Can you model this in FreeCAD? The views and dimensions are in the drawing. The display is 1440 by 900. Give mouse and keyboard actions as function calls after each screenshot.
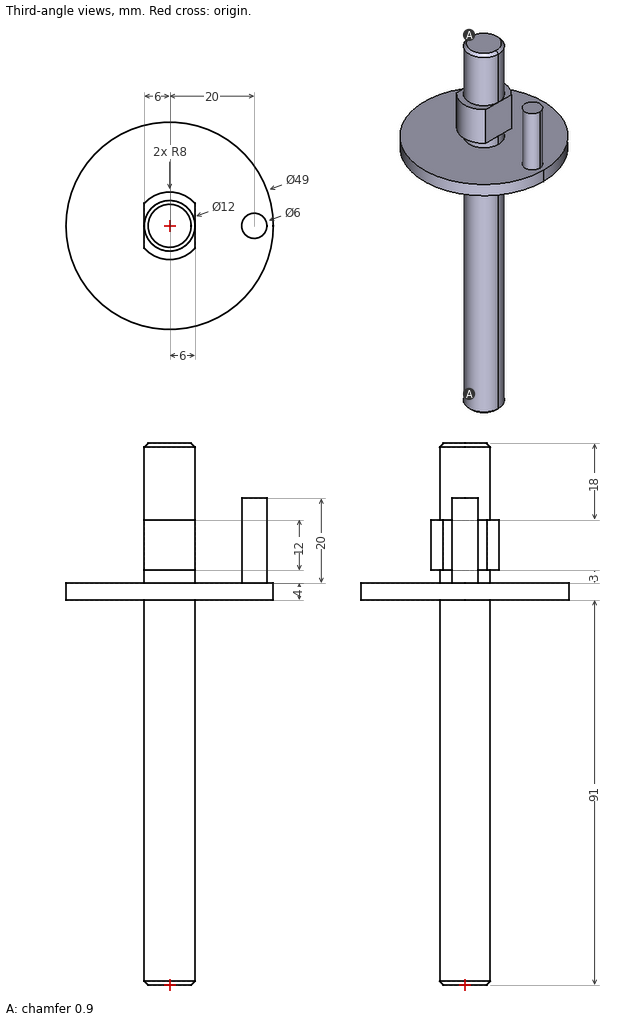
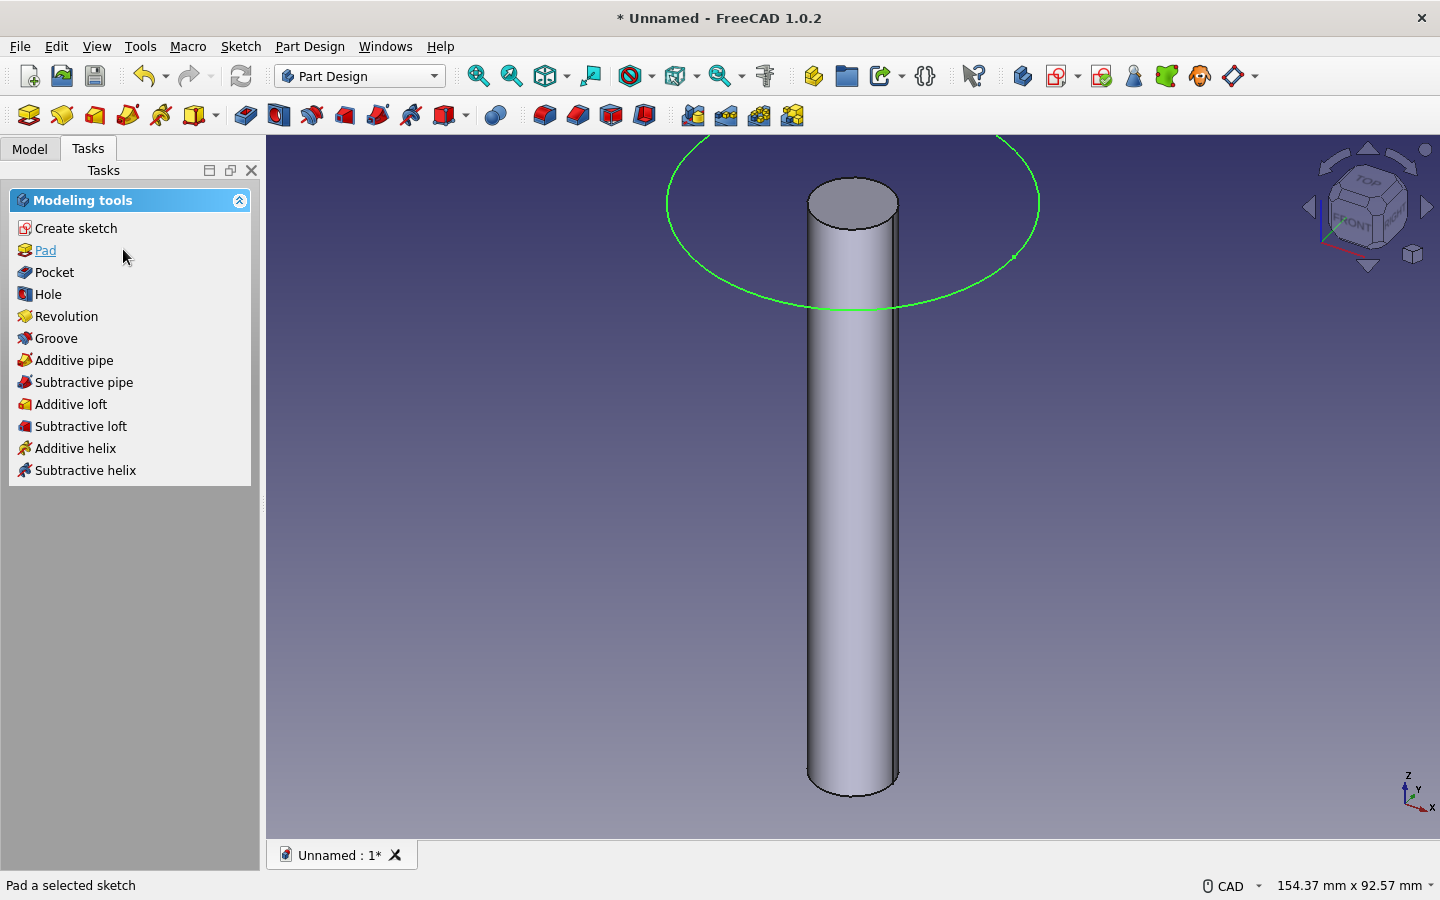
click(29, 116)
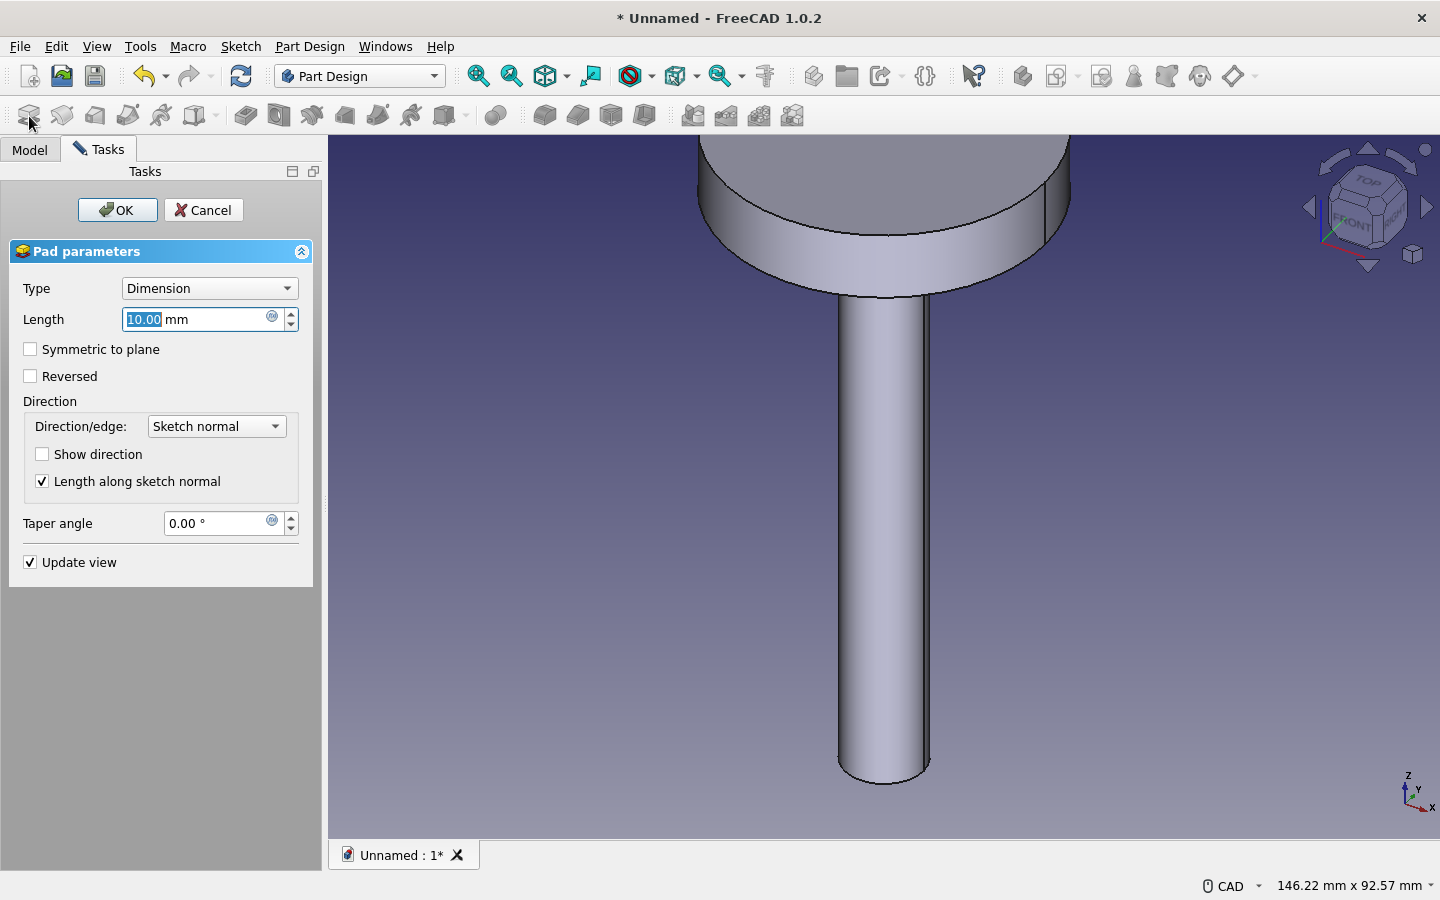
text(4)
key(Tab)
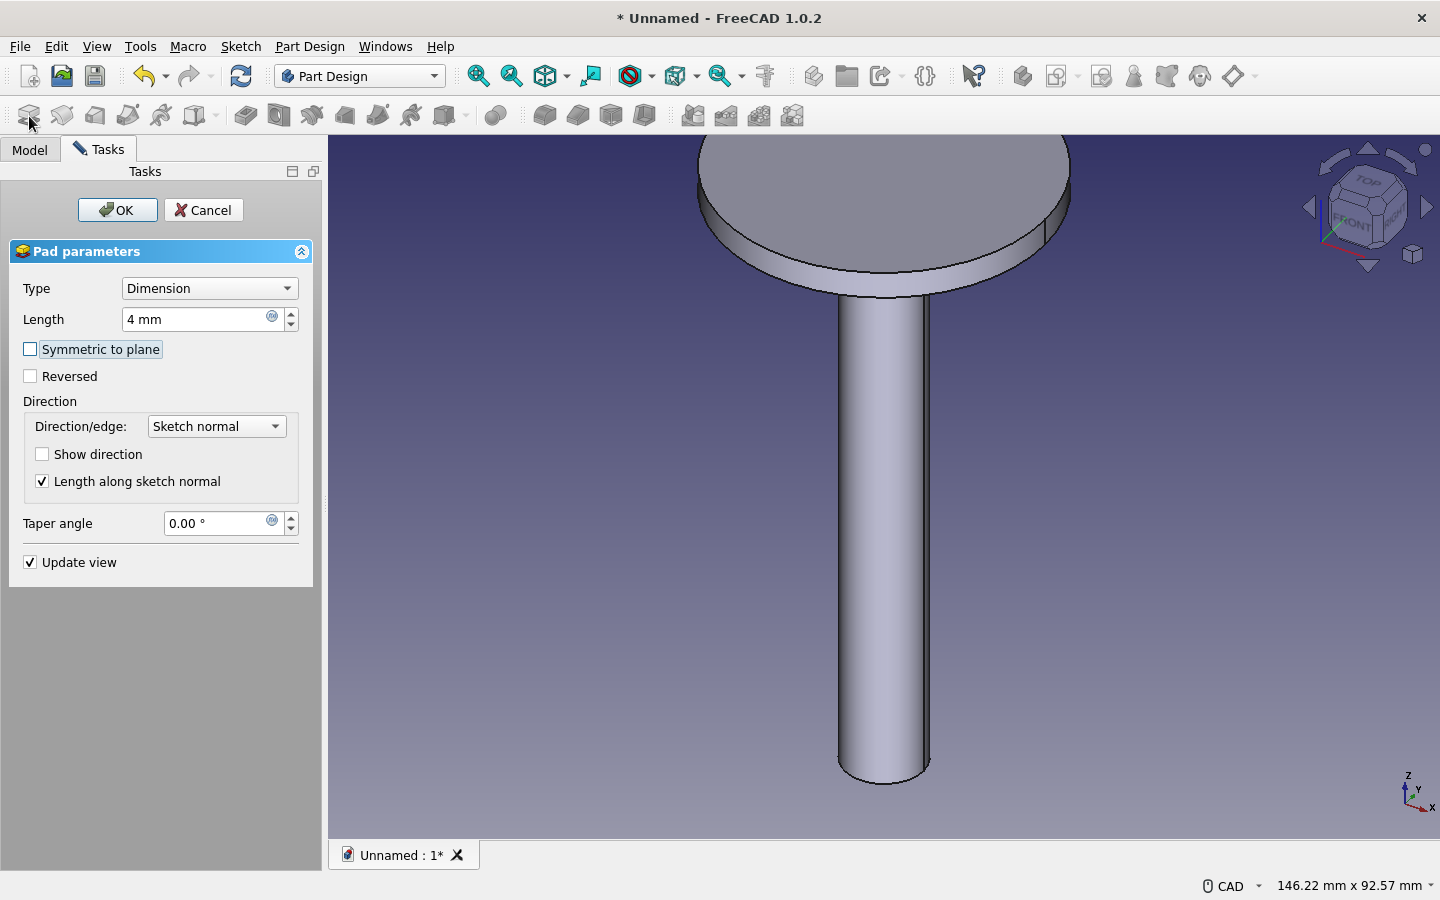
click(118, 210)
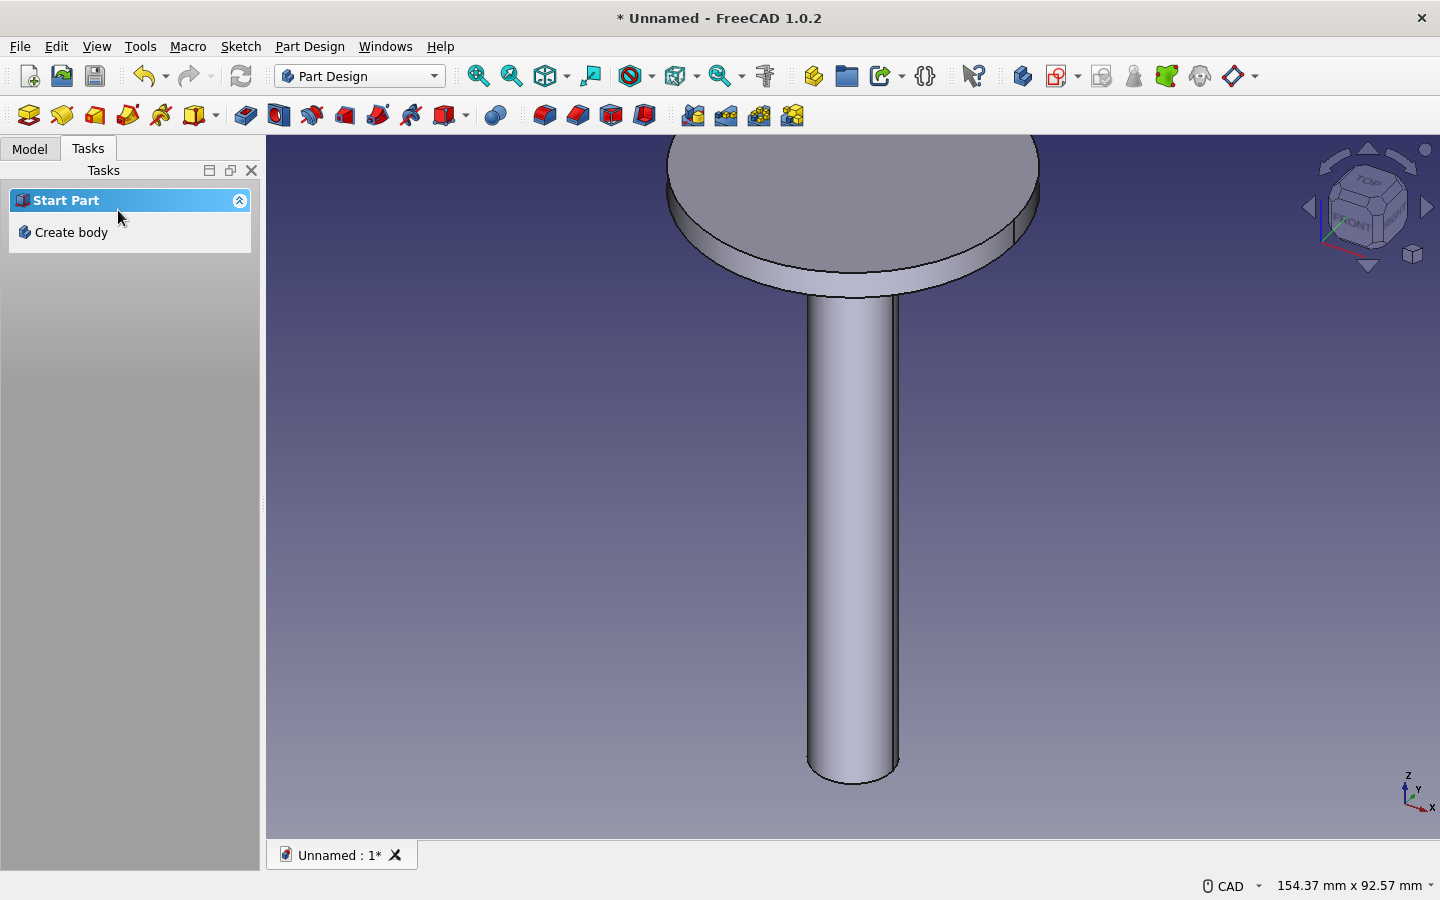
key(v)
key(f)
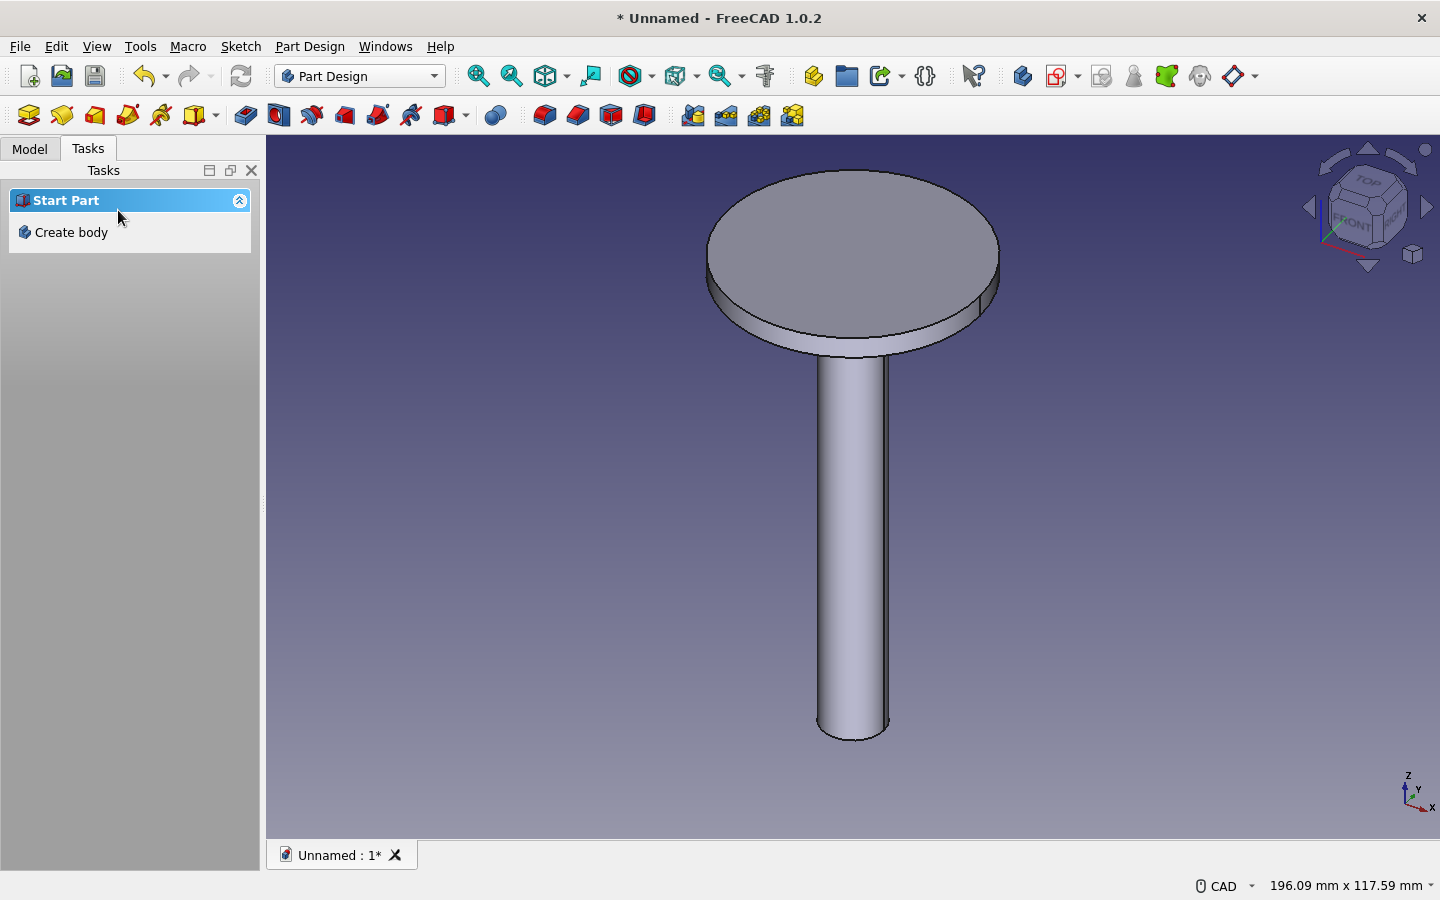
click(853, 253)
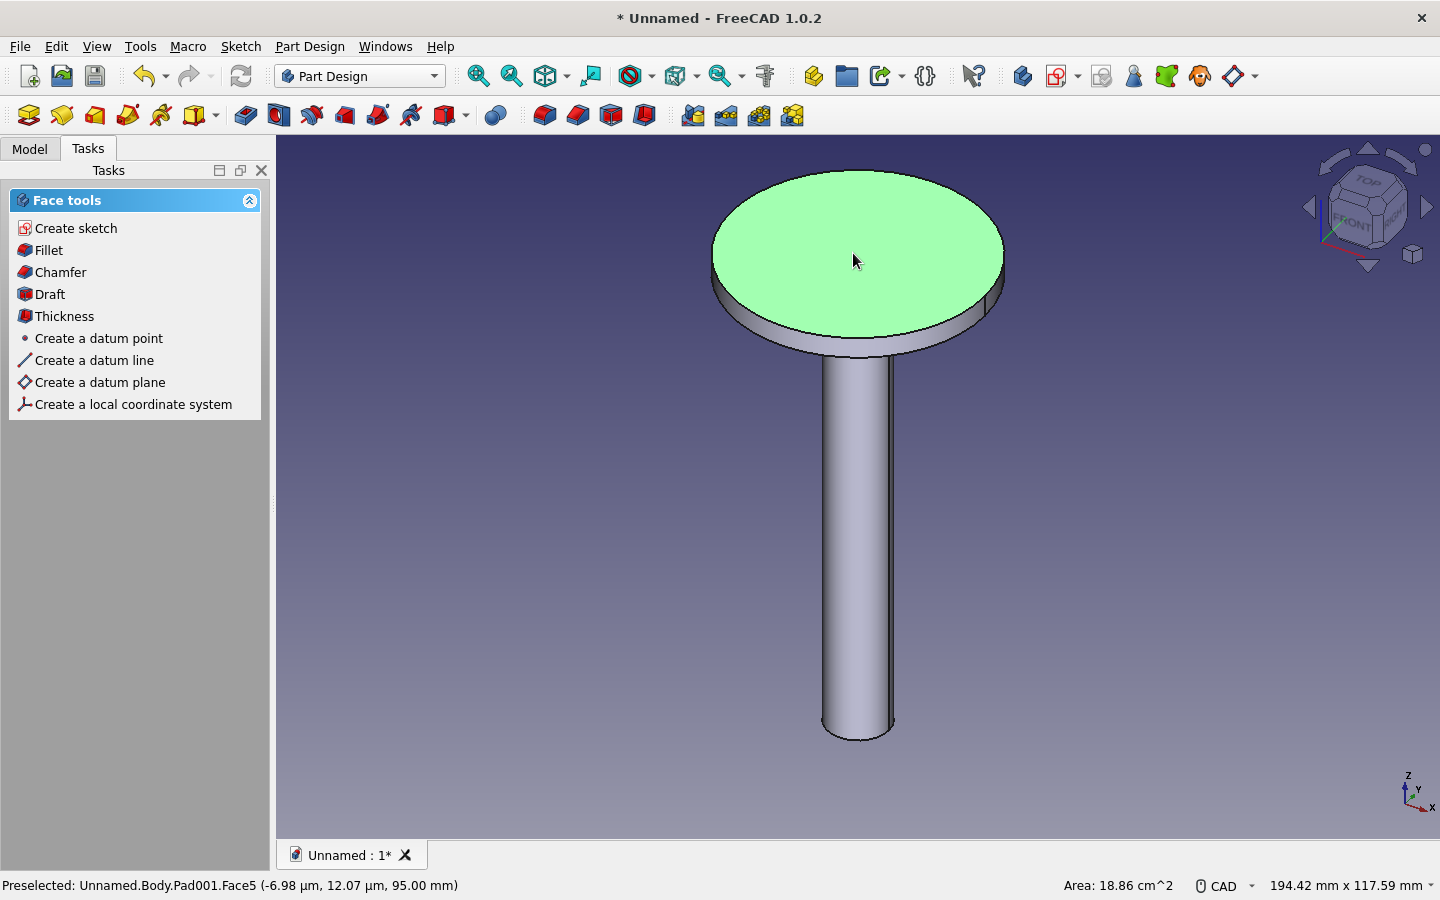
click(1056, 76)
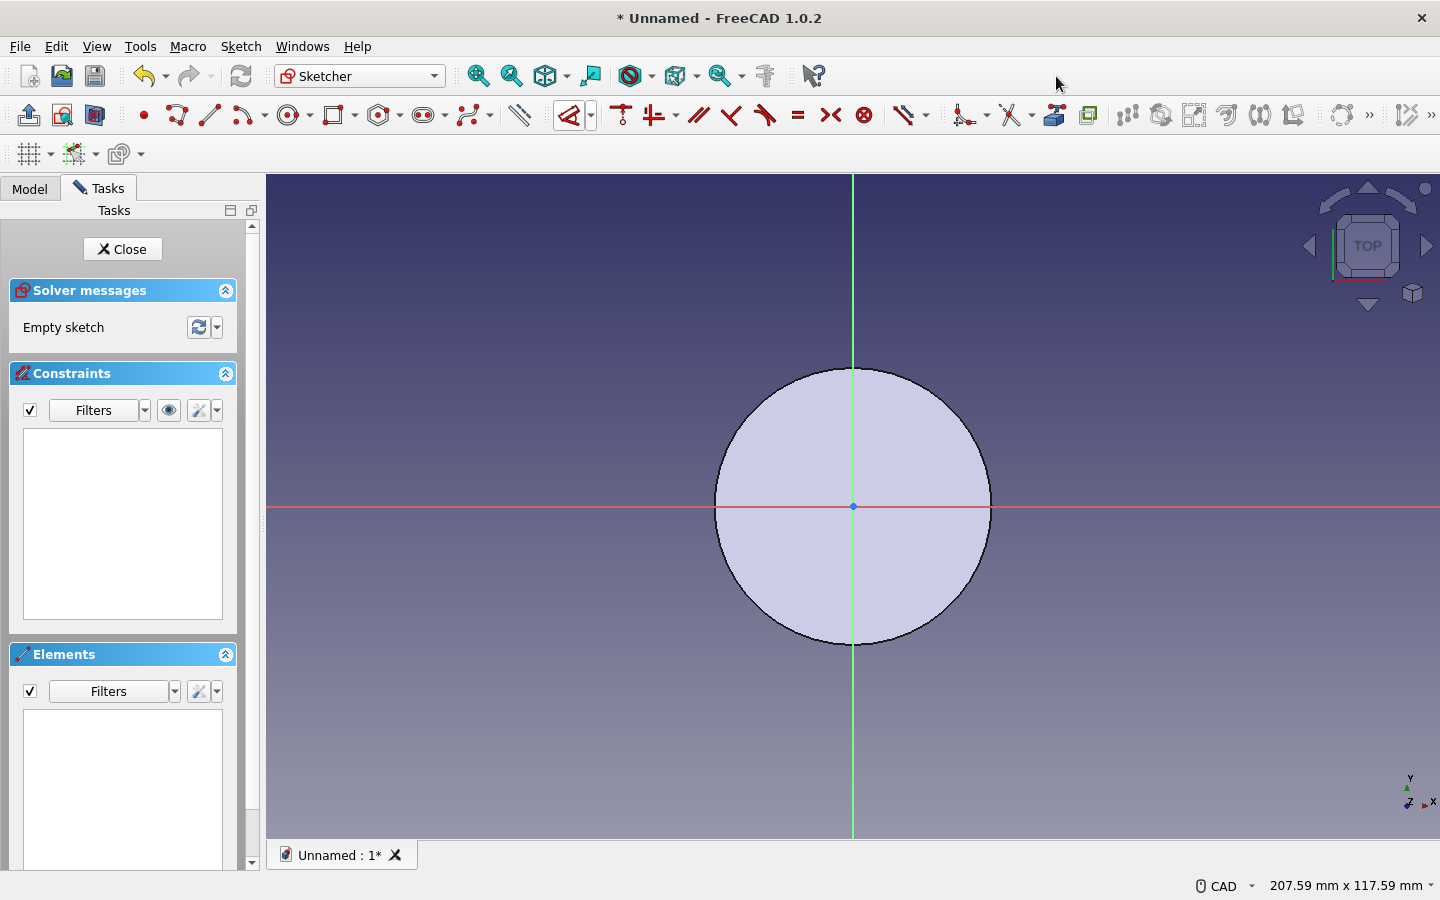
scroll(867, 506, up, 9)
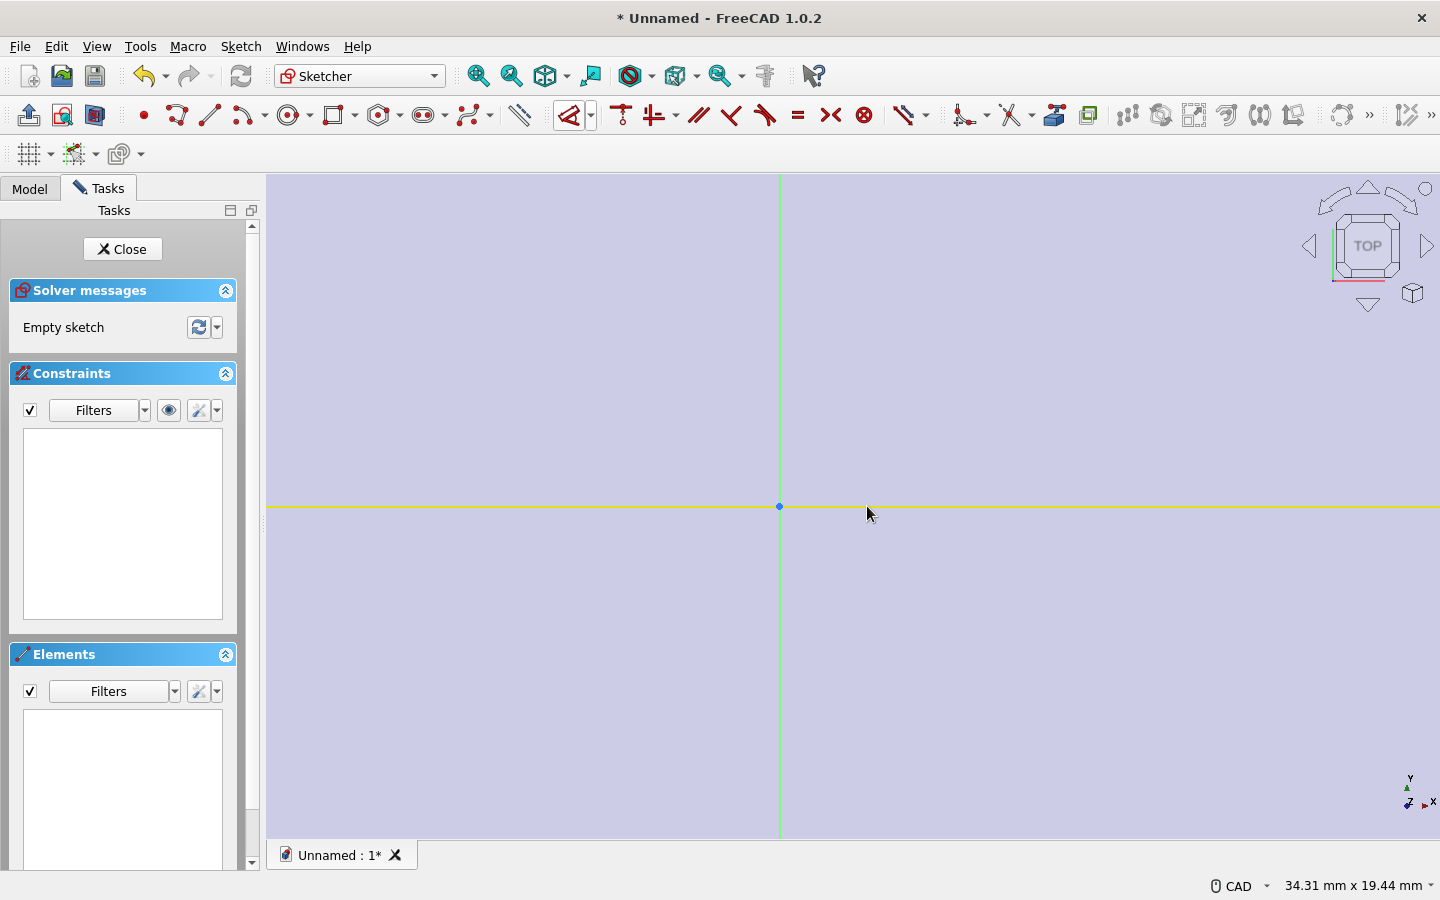
key(g)
key(c)